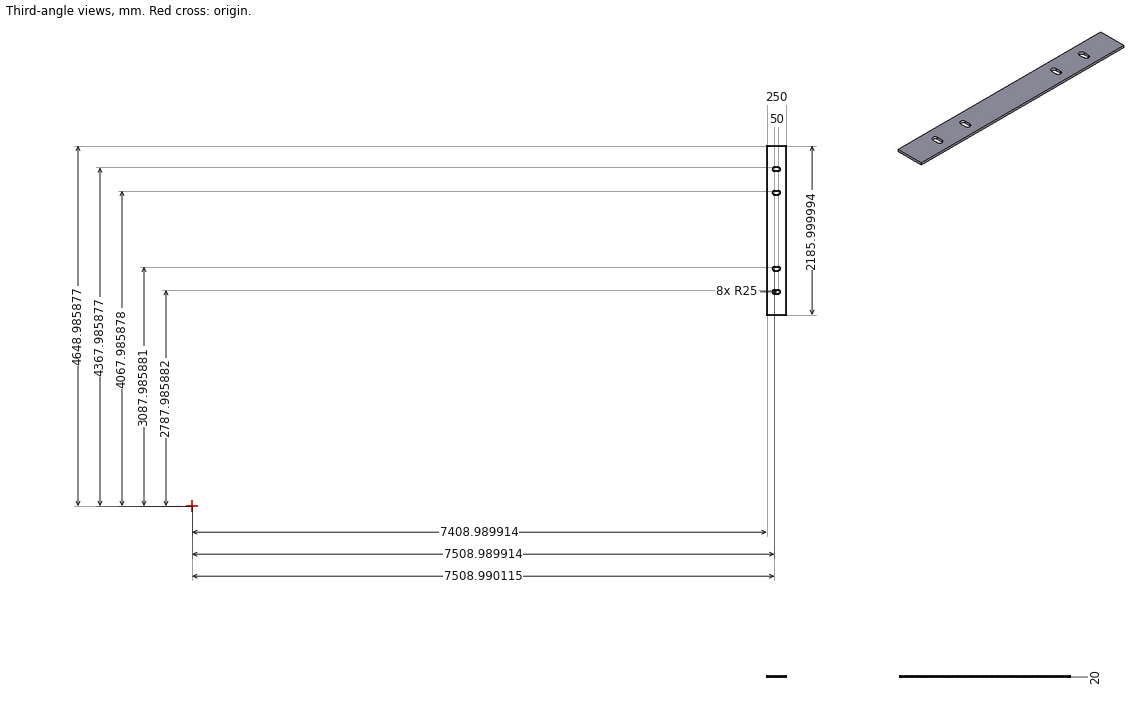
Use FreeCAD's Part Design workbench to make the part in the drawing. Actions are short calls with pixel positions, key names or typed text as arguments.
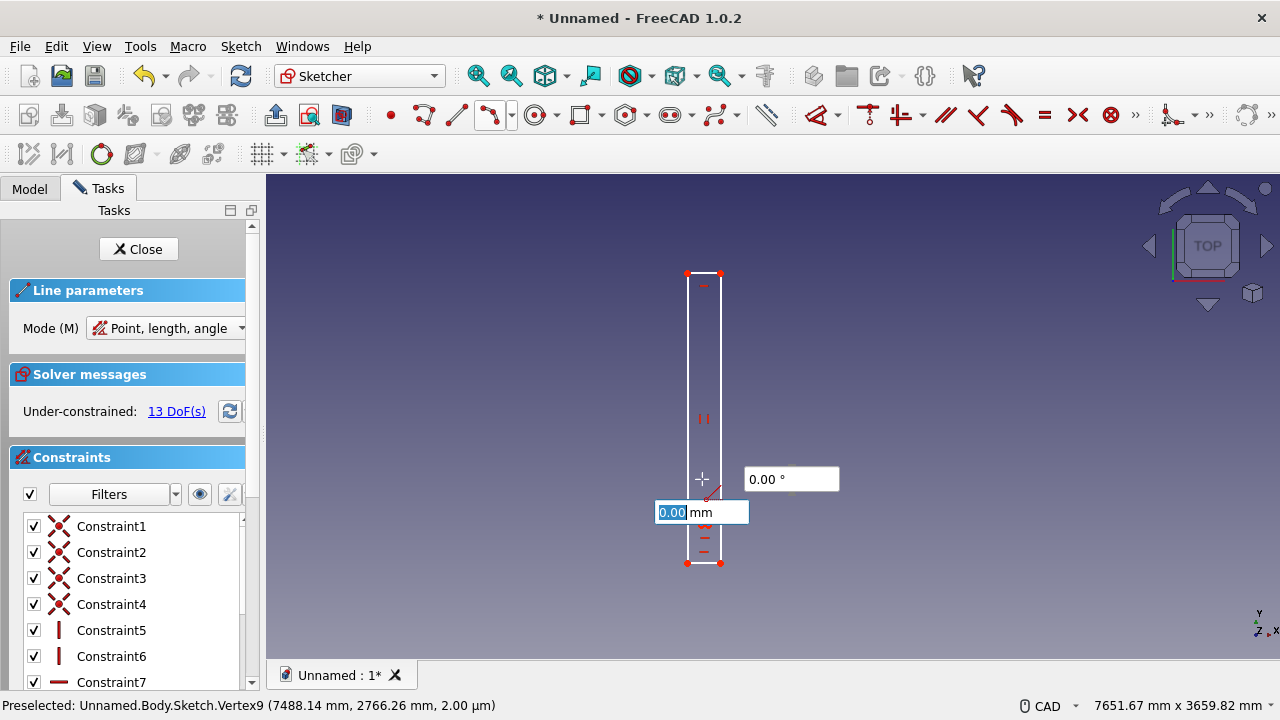
scroll(708, 479, up, 5)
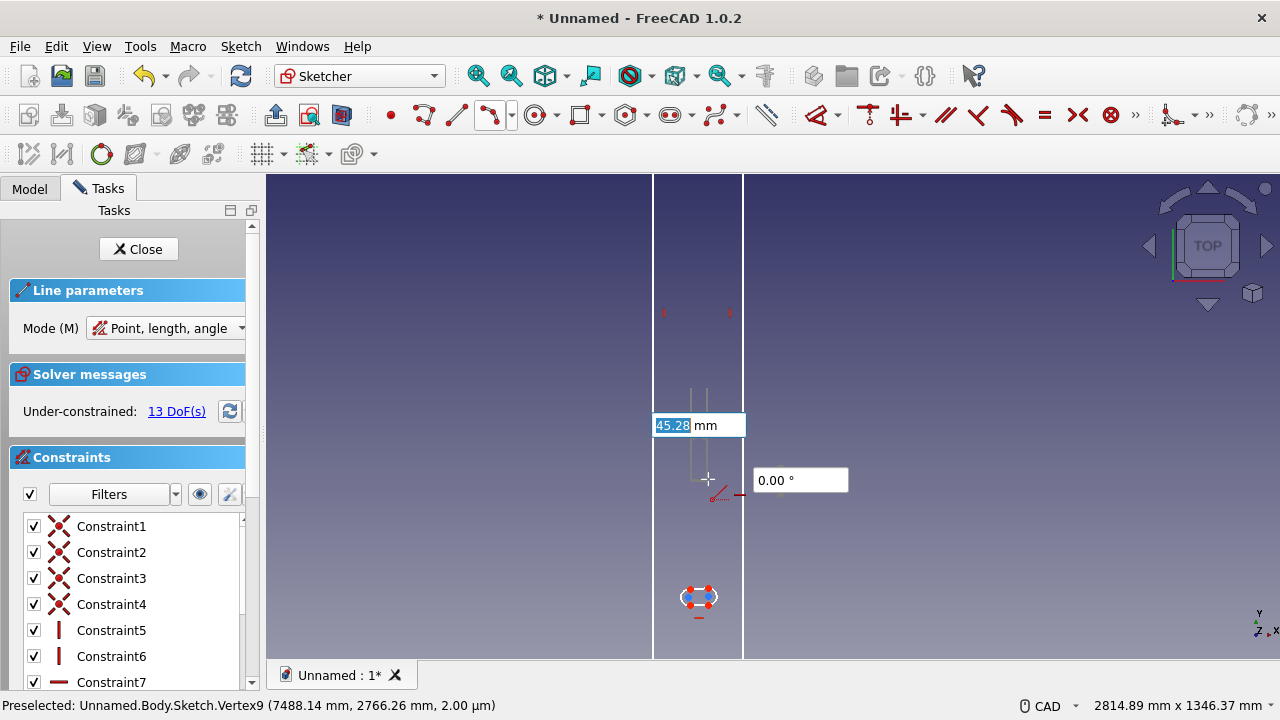
click(708, 478)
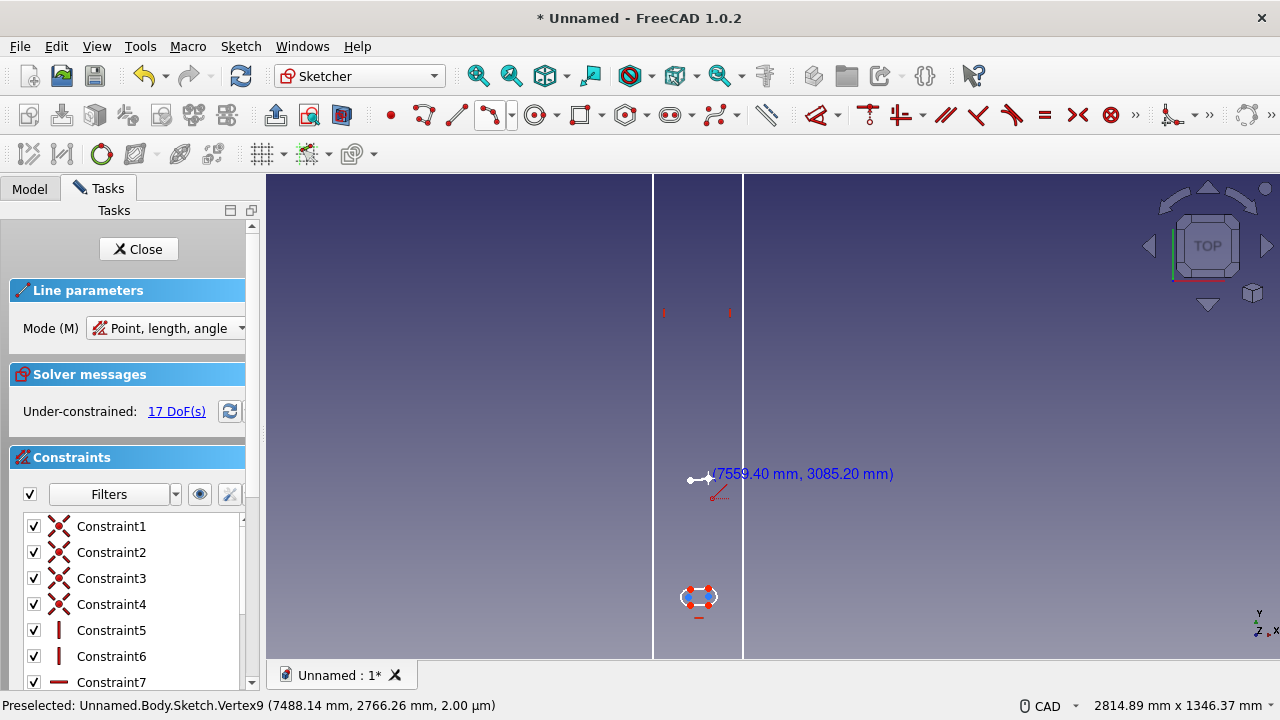
click(708, 496)
click(690, 496)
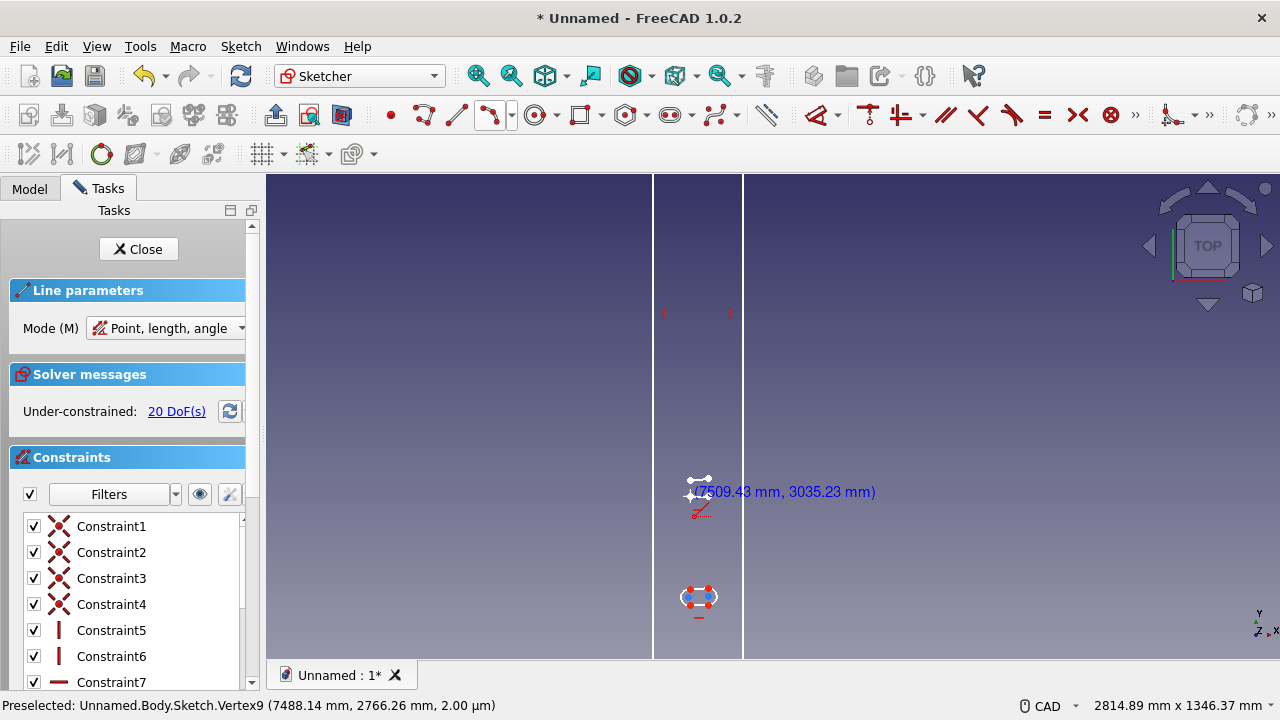
key(g)
key(3)
key(a)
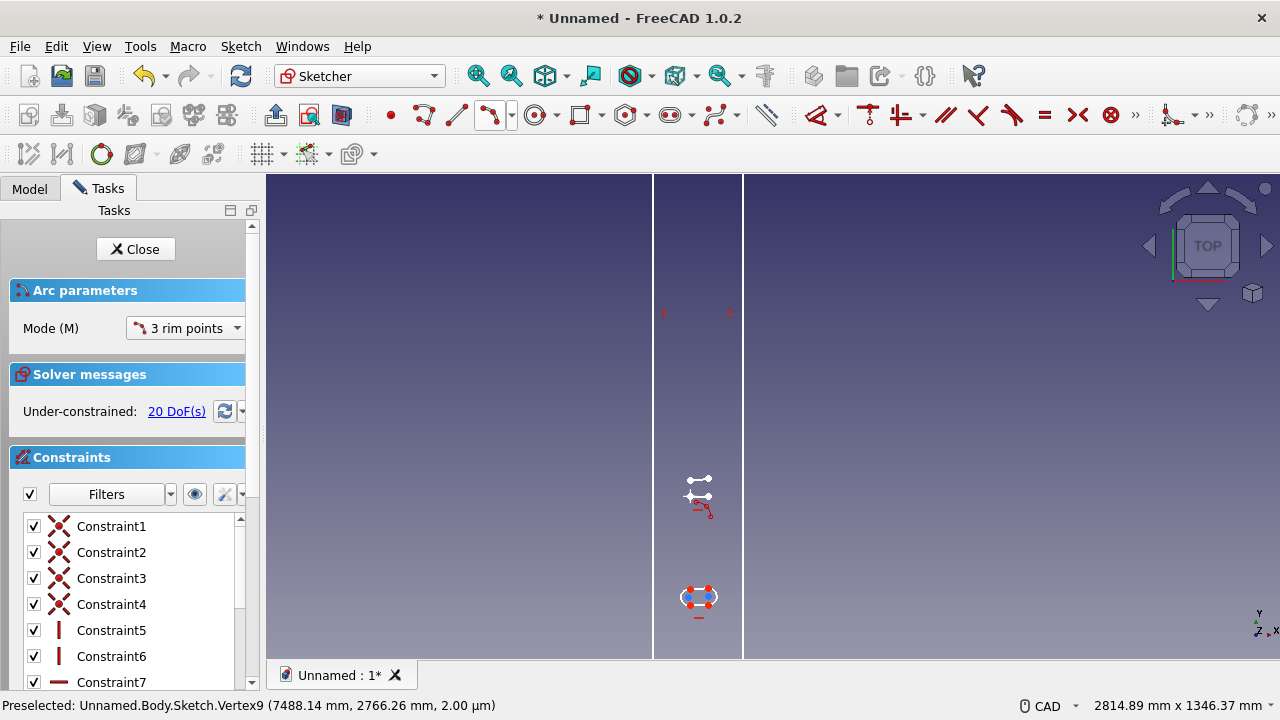
scroll(708, 478, up, 3)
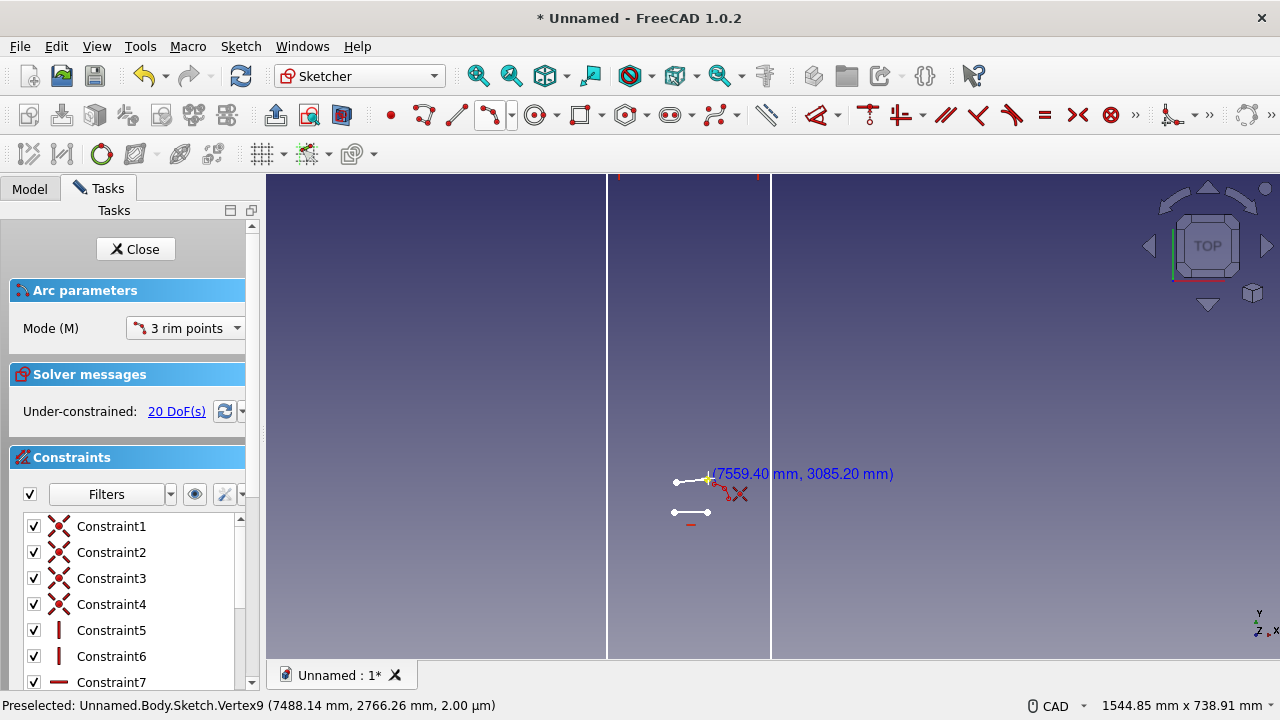
click(708, 479)
click(708, 512)
click(724, 494)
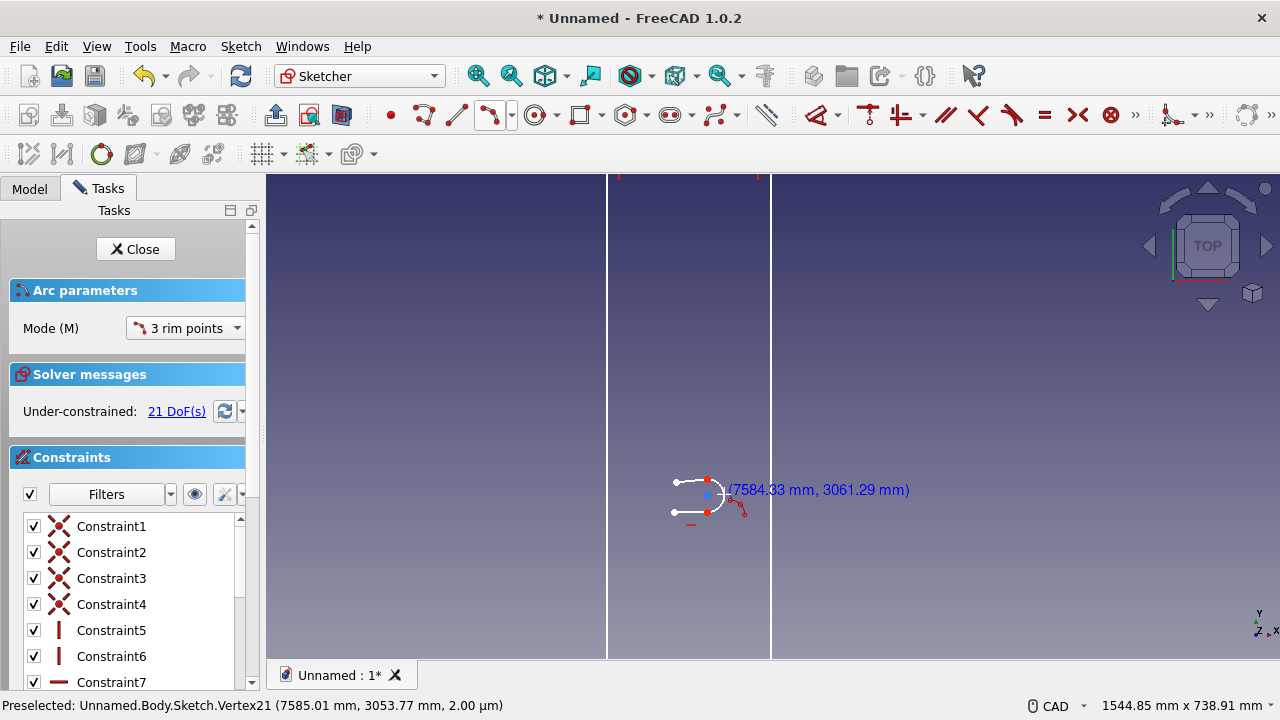
click(675, 512)
click(677, 482)
click(658, 494)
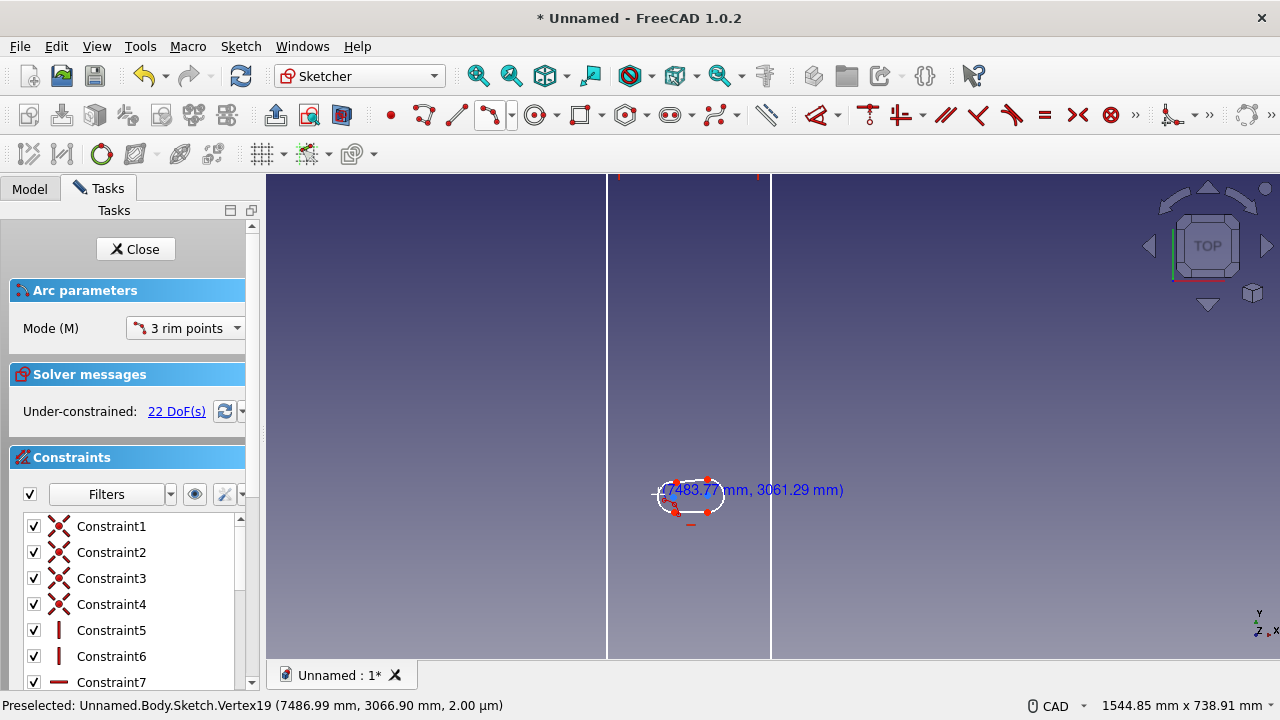
key(g)
key(l)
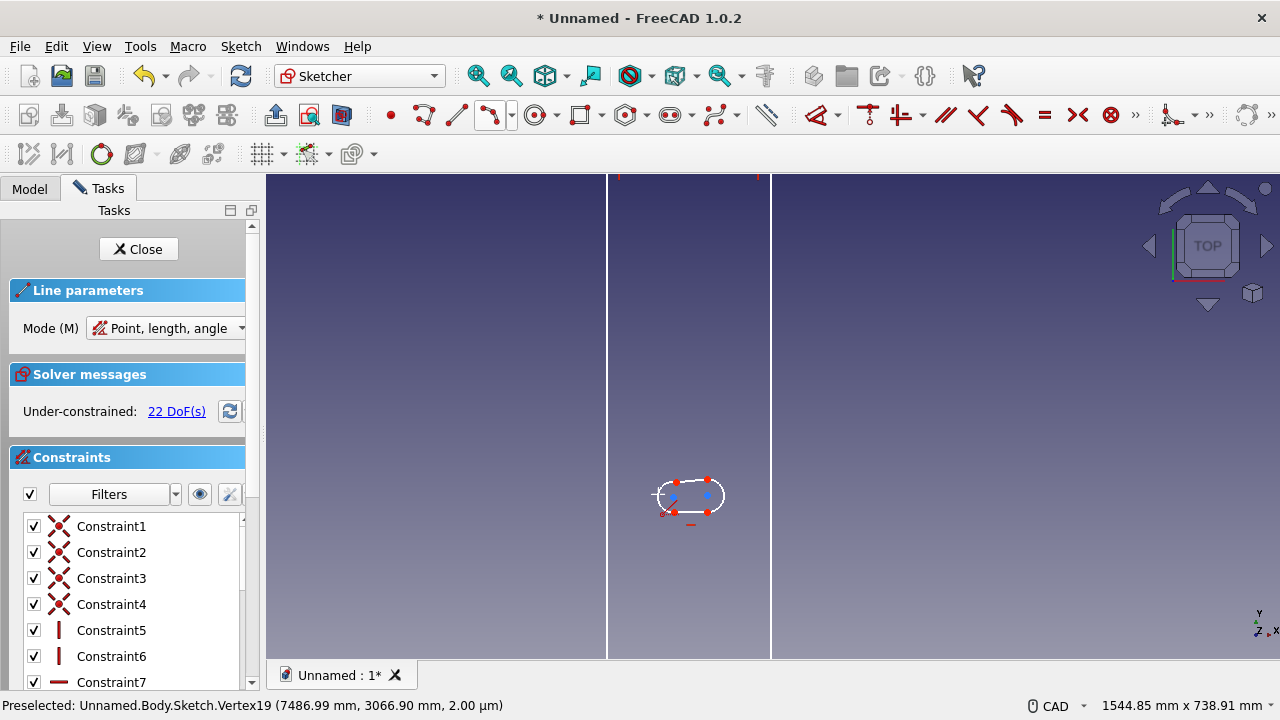
scroll(708, 479, down, 8)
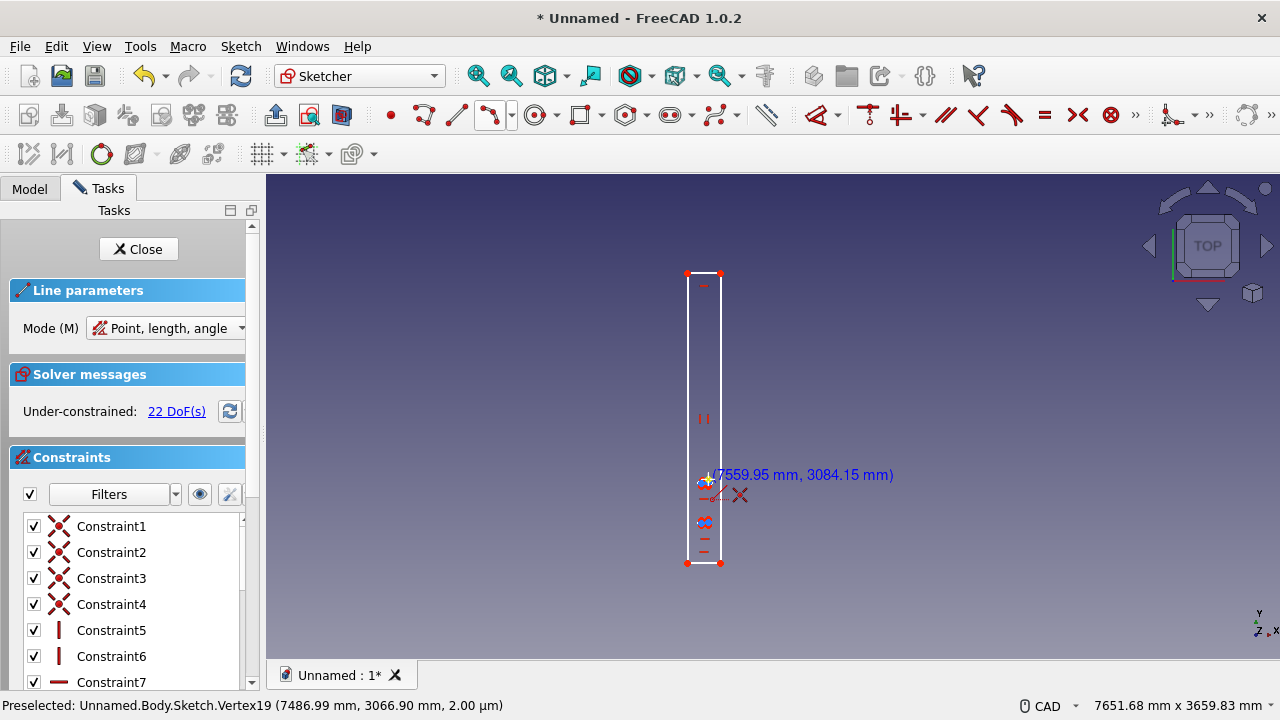
click(702, 310)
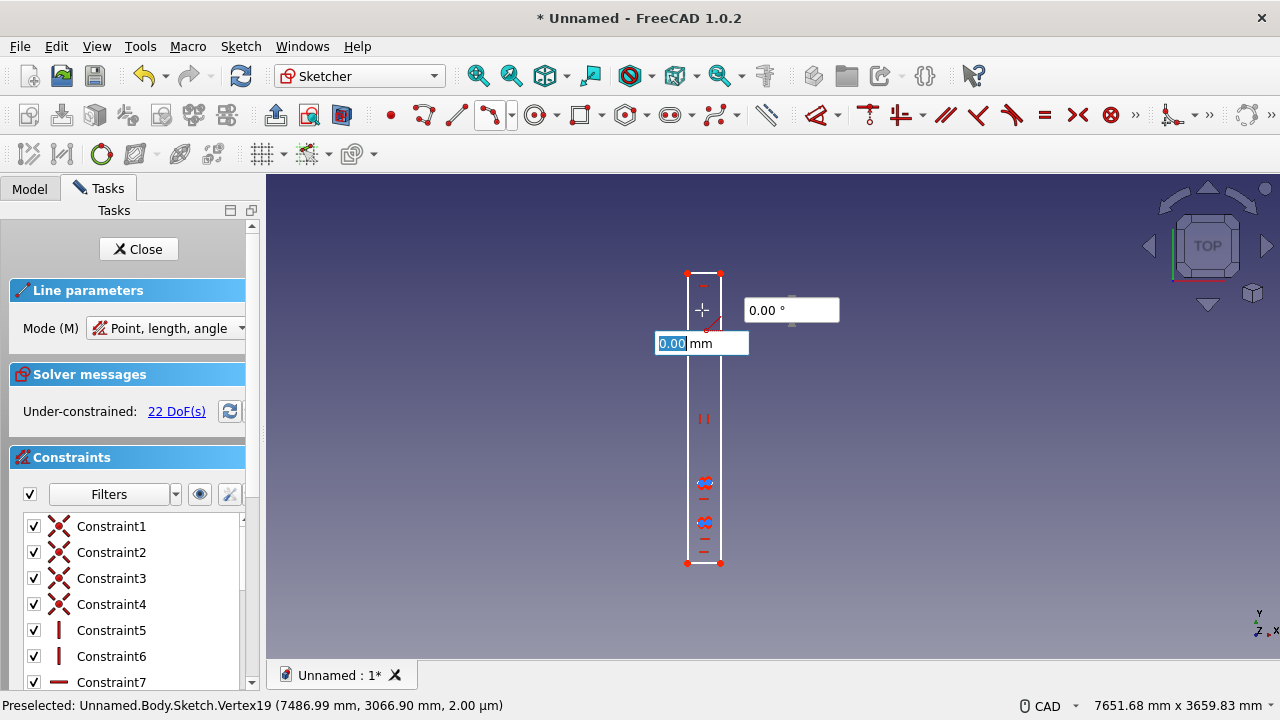
scroll(708, 310, up, 5)